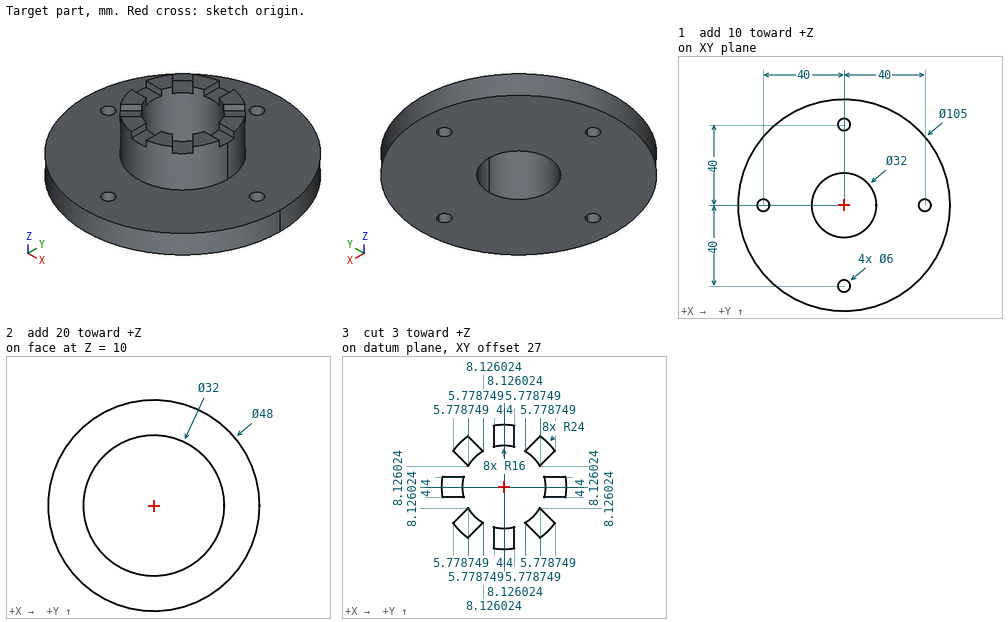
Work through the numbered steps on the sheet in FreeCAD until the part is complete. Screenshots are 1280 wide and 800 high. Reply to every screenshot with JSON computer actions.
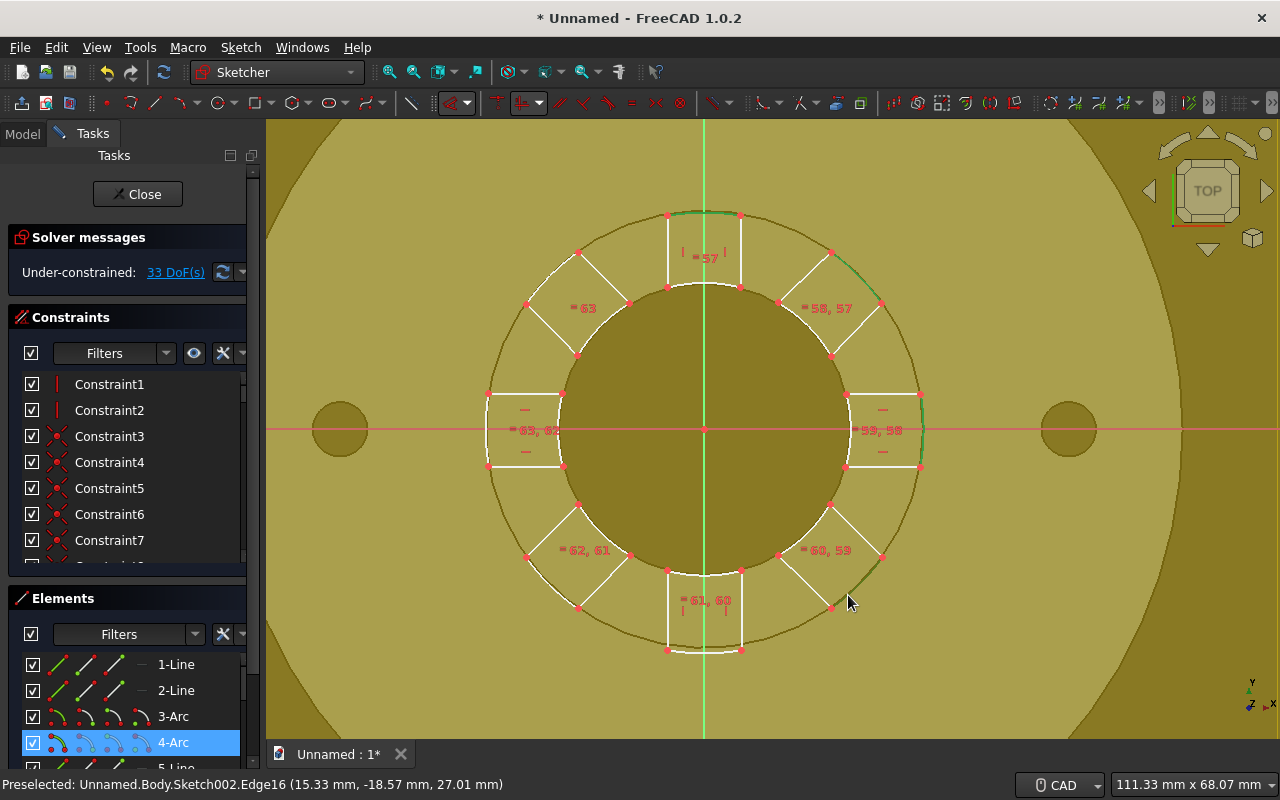
{"action": "left_click", "coordinate": [690, 653]}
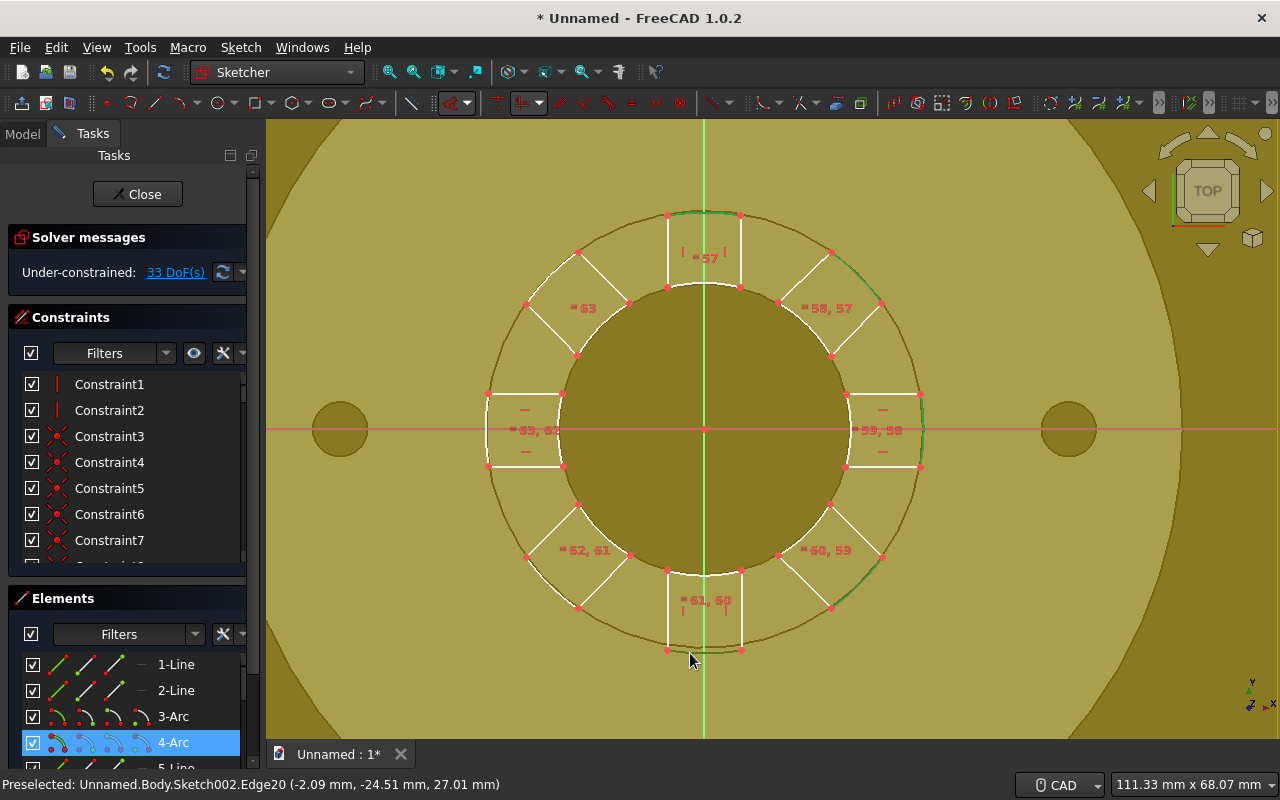
{"action": "left_click", "coordinate": [540, 575]}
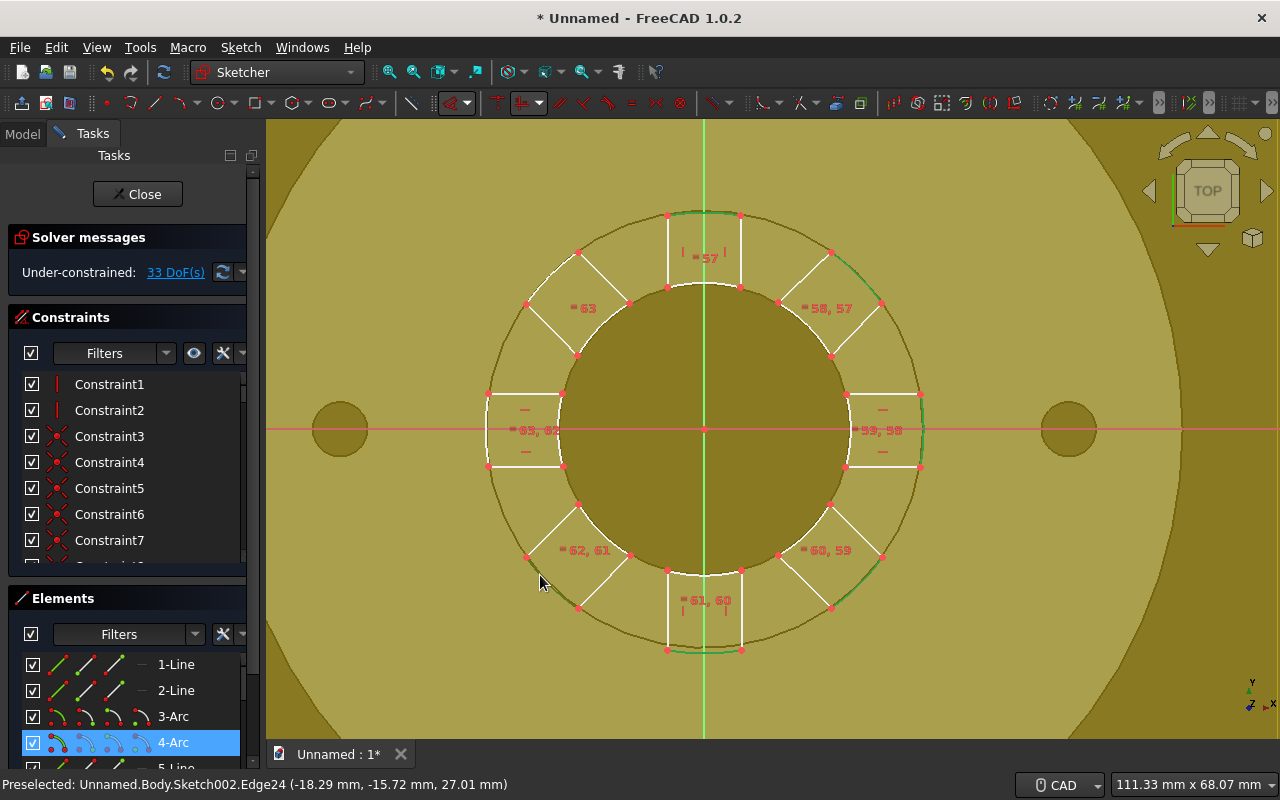
{"action": "left_click", "coordinate": [486, 416]}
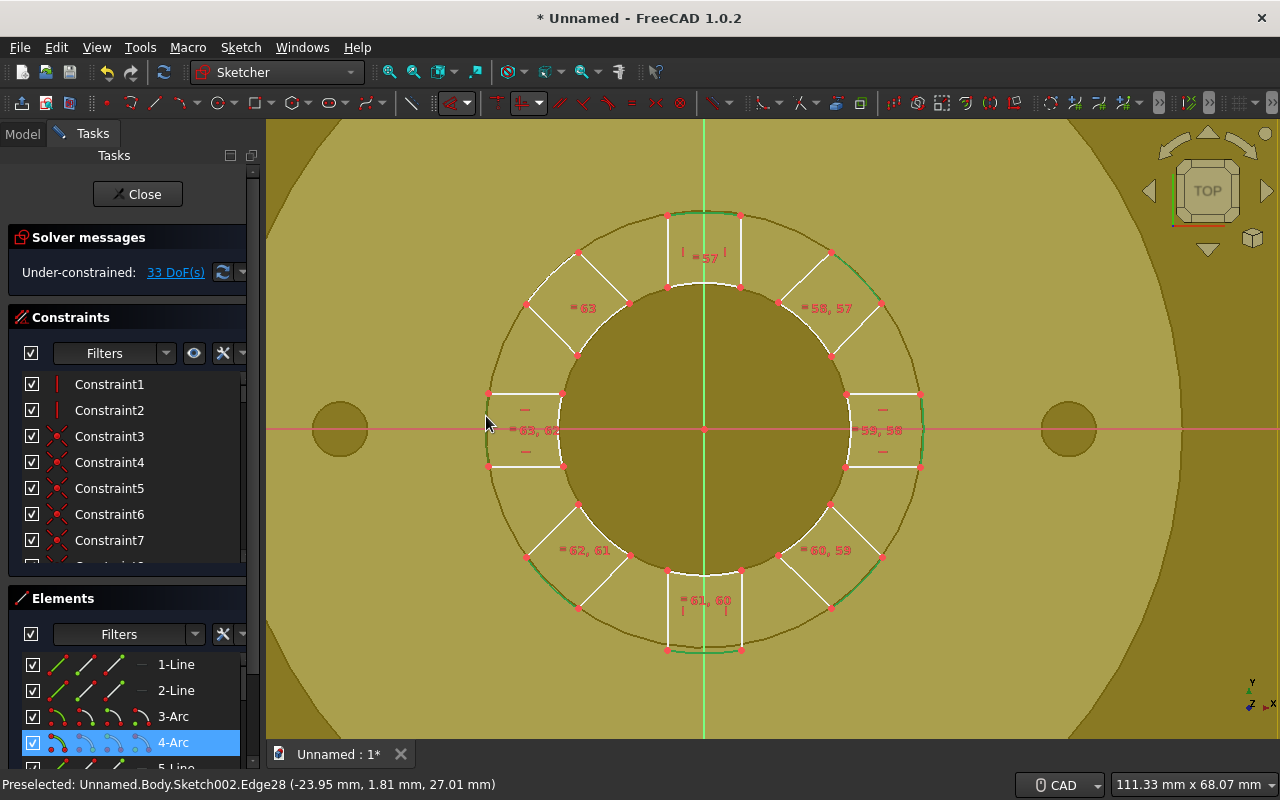
{"action": "left_click", "coordinate": [561, 266]}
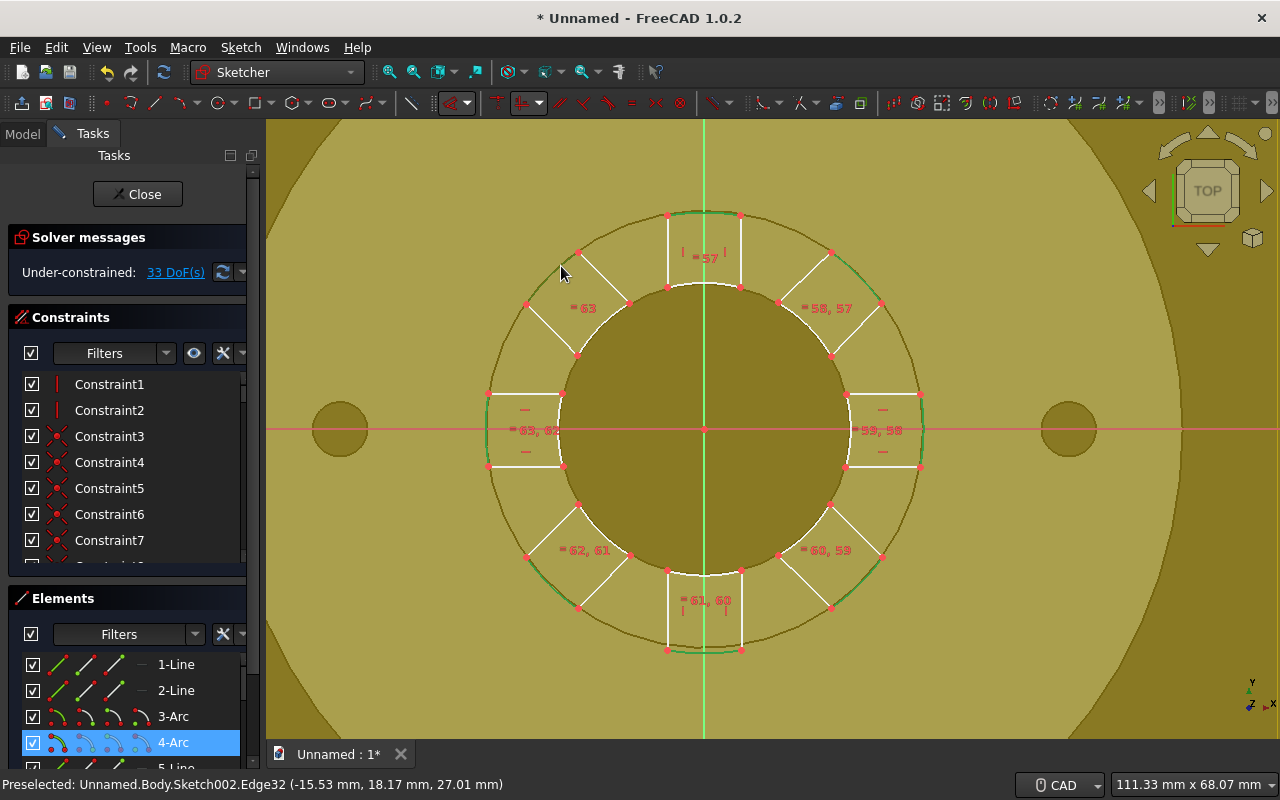
{"action": "left_click", "coordinate": [632, 104]}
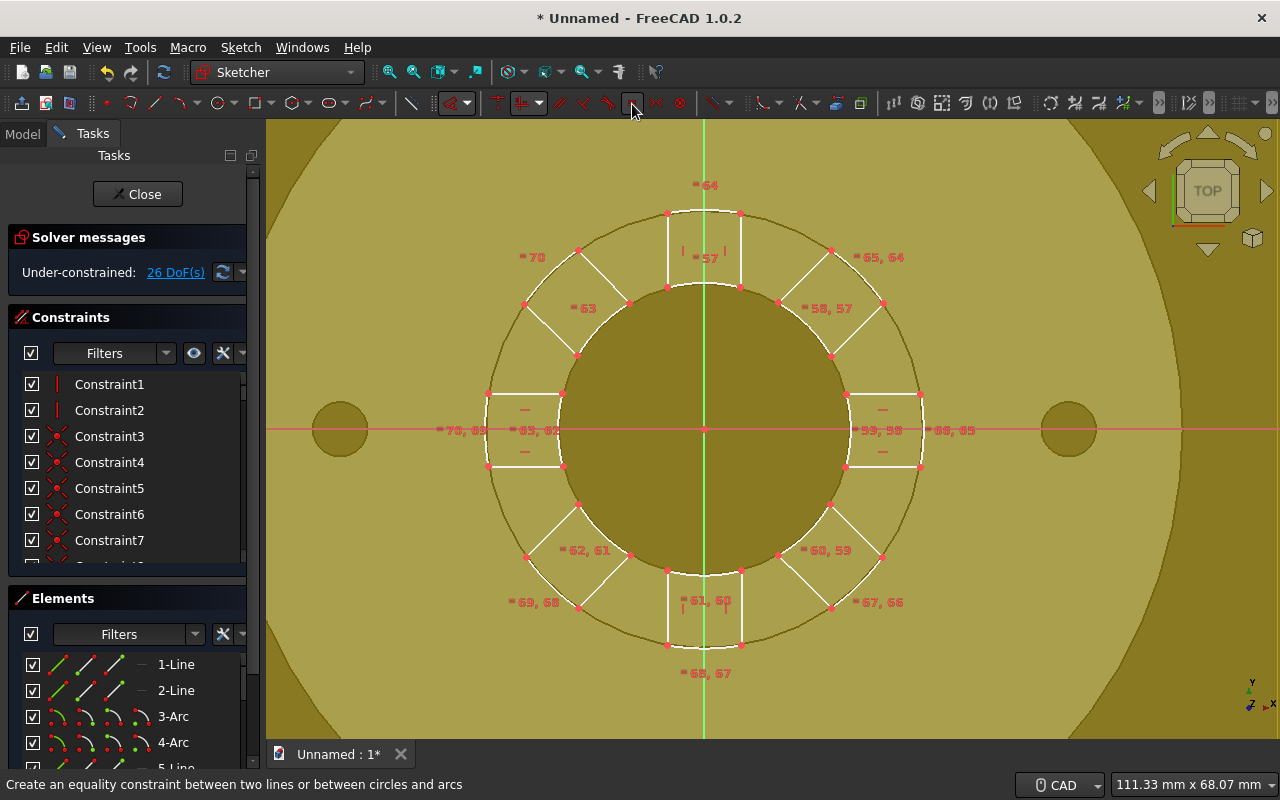
{"action": "left_click", "coordinate": [719, 284]}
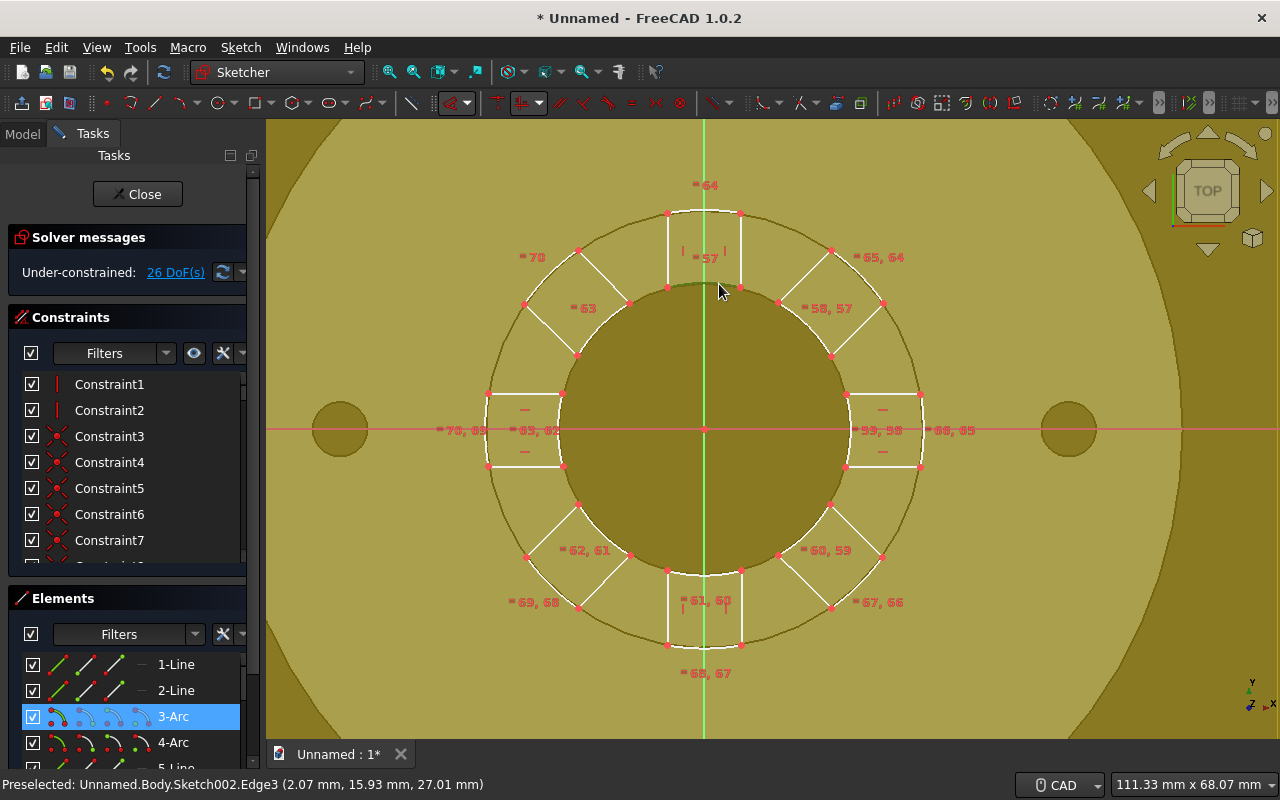
{"action": "left_click", "coordinate": [470, 104]}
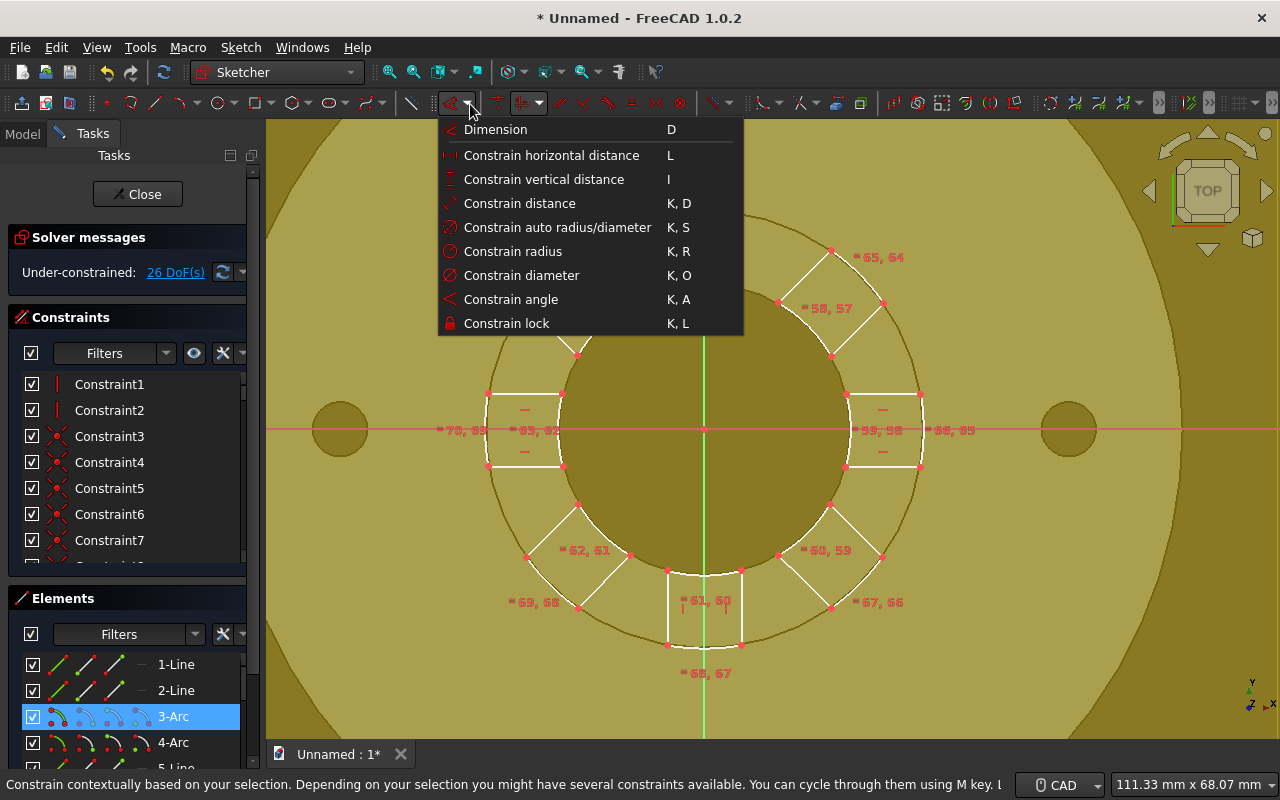
{"action": "left_click", "coordinate": [591, 251]}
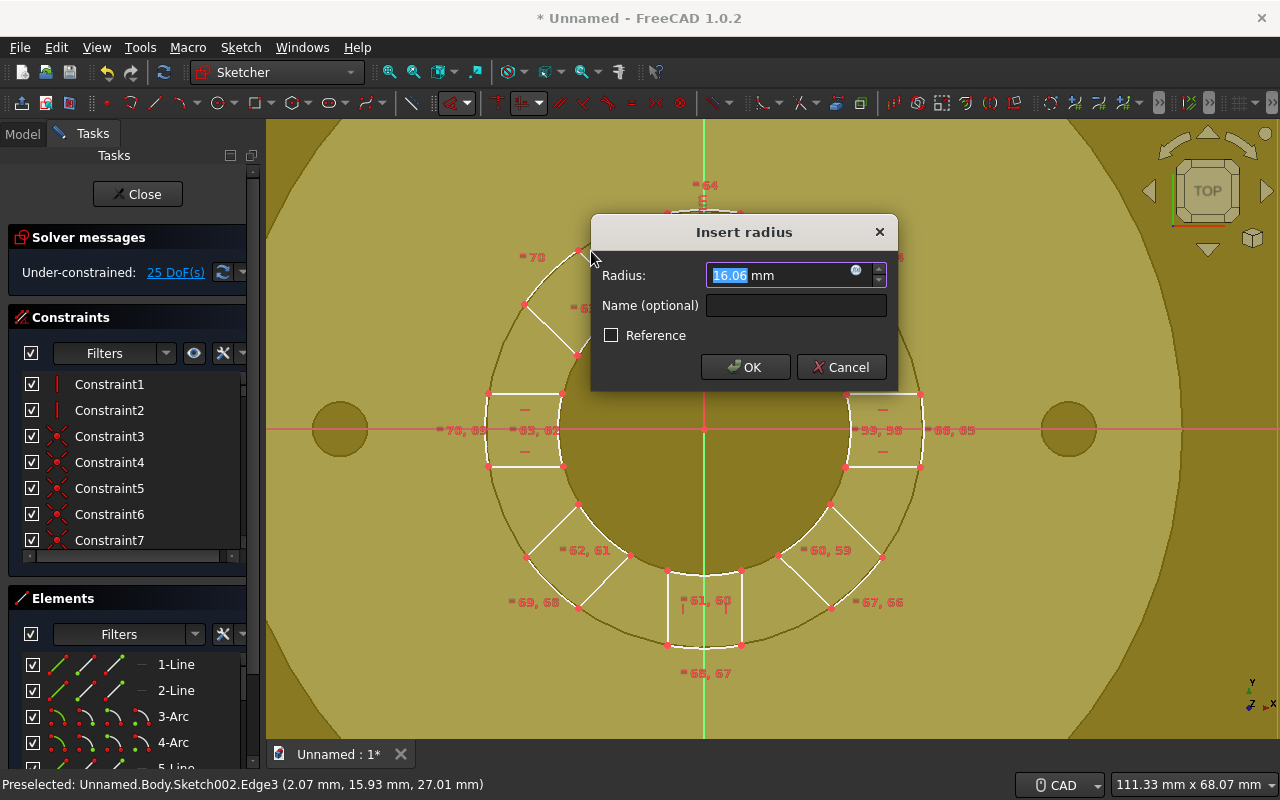
{"action": "type", "text": "16"}
{"action": "key", "text": "Return"}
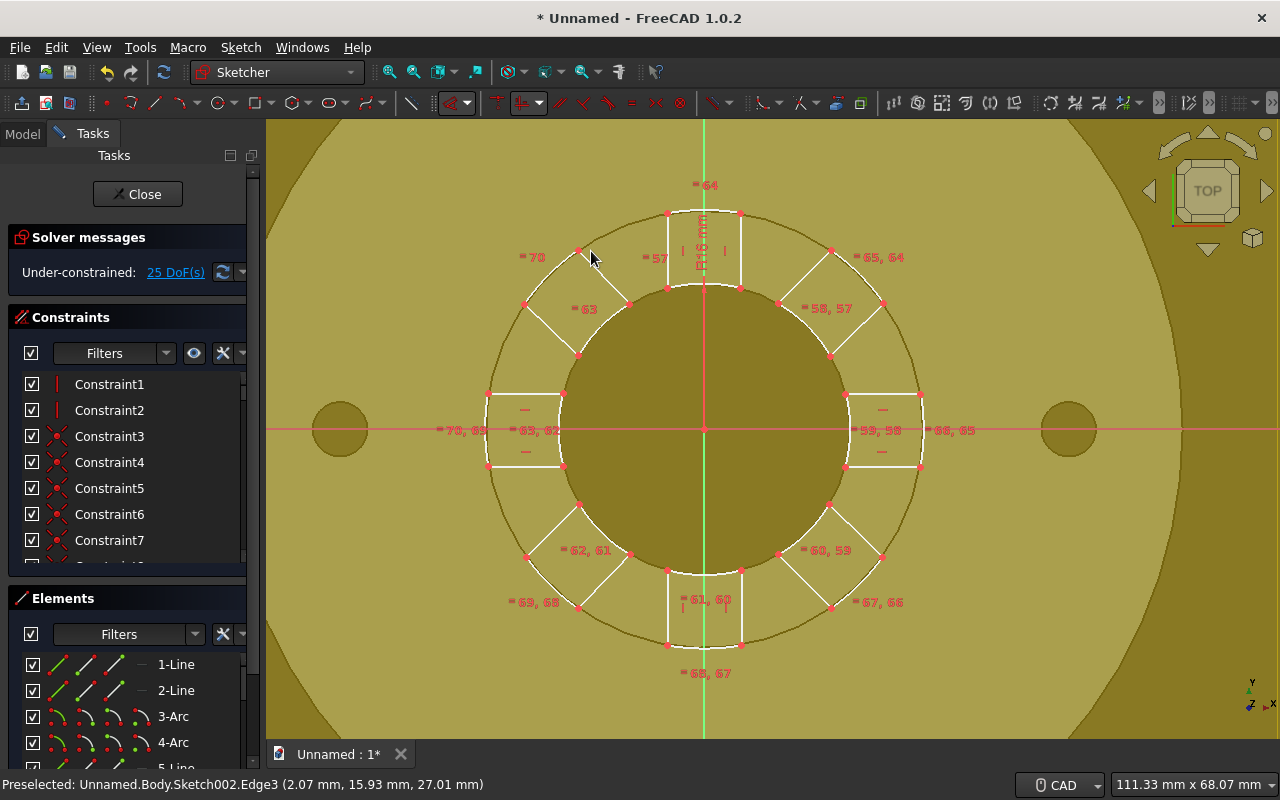
{"action": "left_click", "coordinate": [719, 211]}